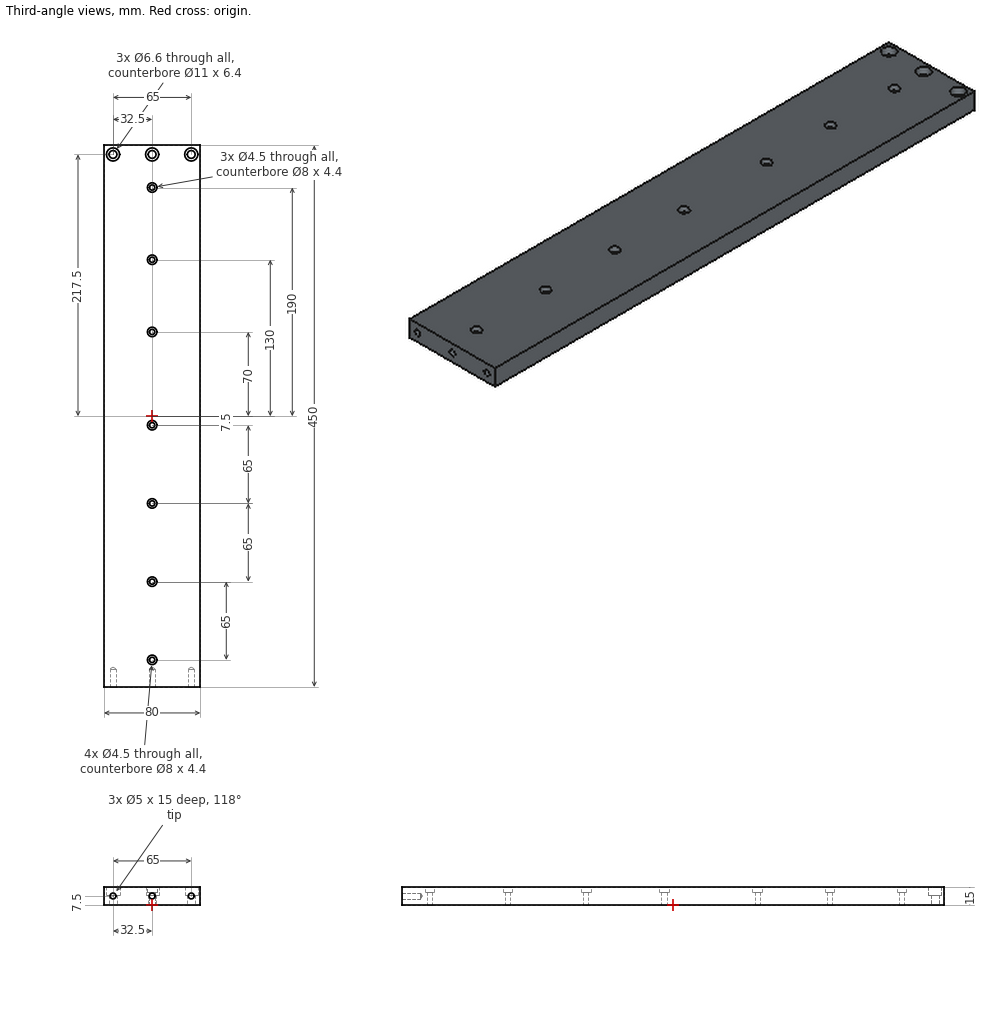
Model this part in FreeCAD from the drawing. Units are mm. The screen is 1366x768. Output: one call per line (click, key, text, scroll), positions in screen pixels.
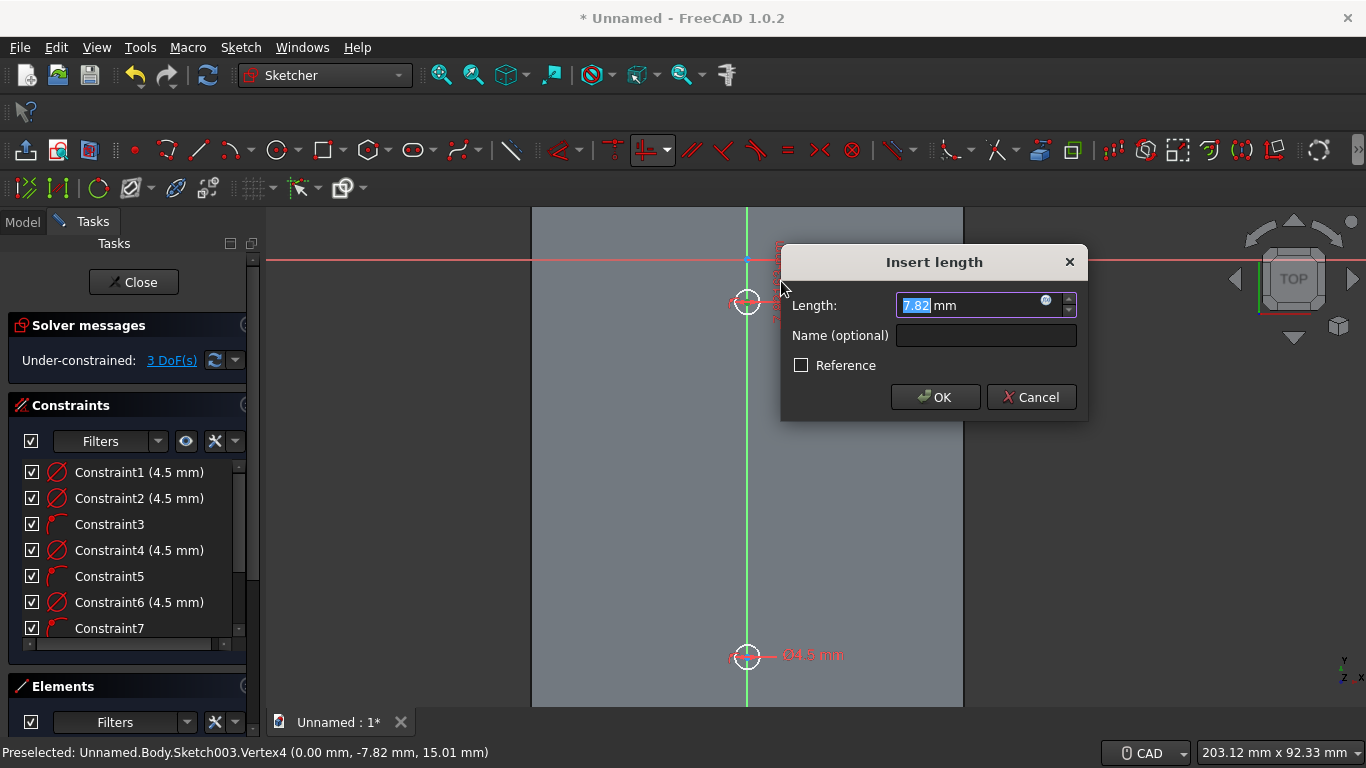
text(7.5)
key(Return)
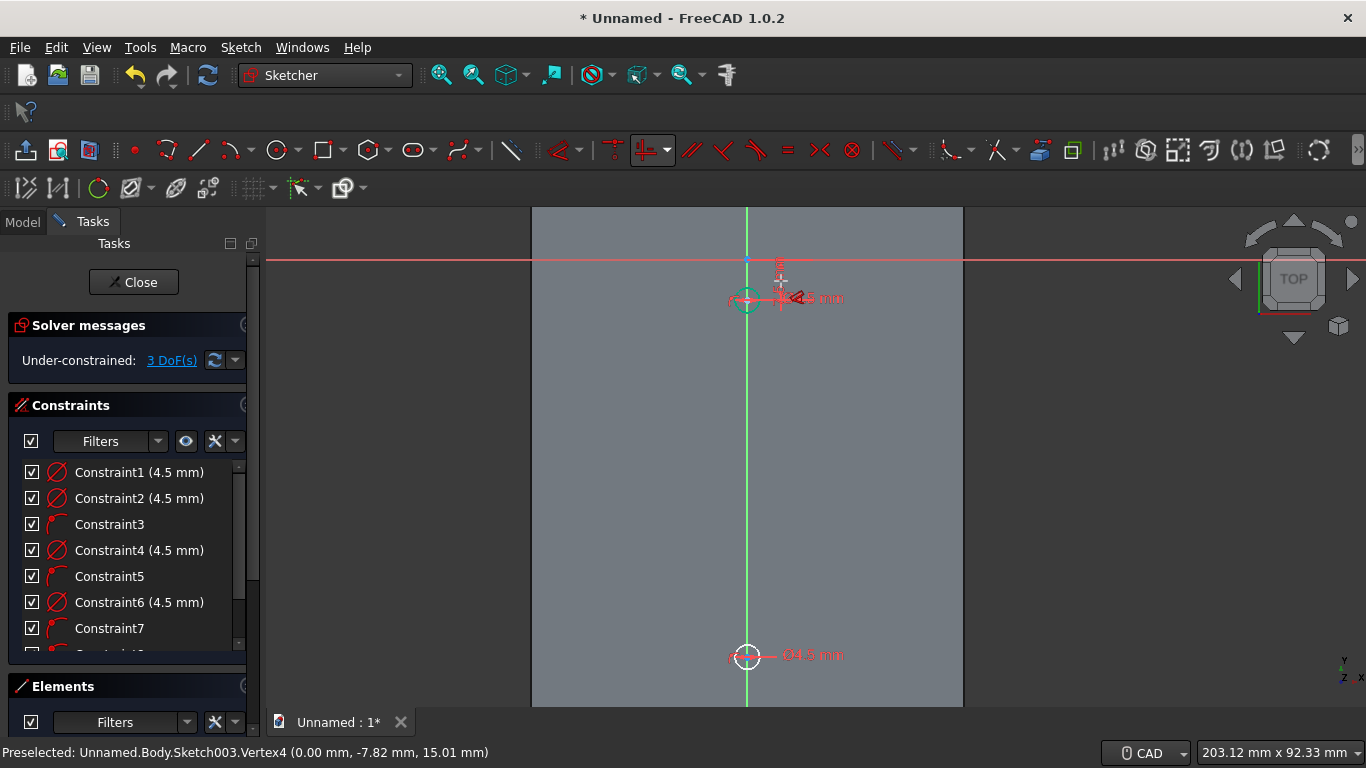
scroll(748, 303, down, 6)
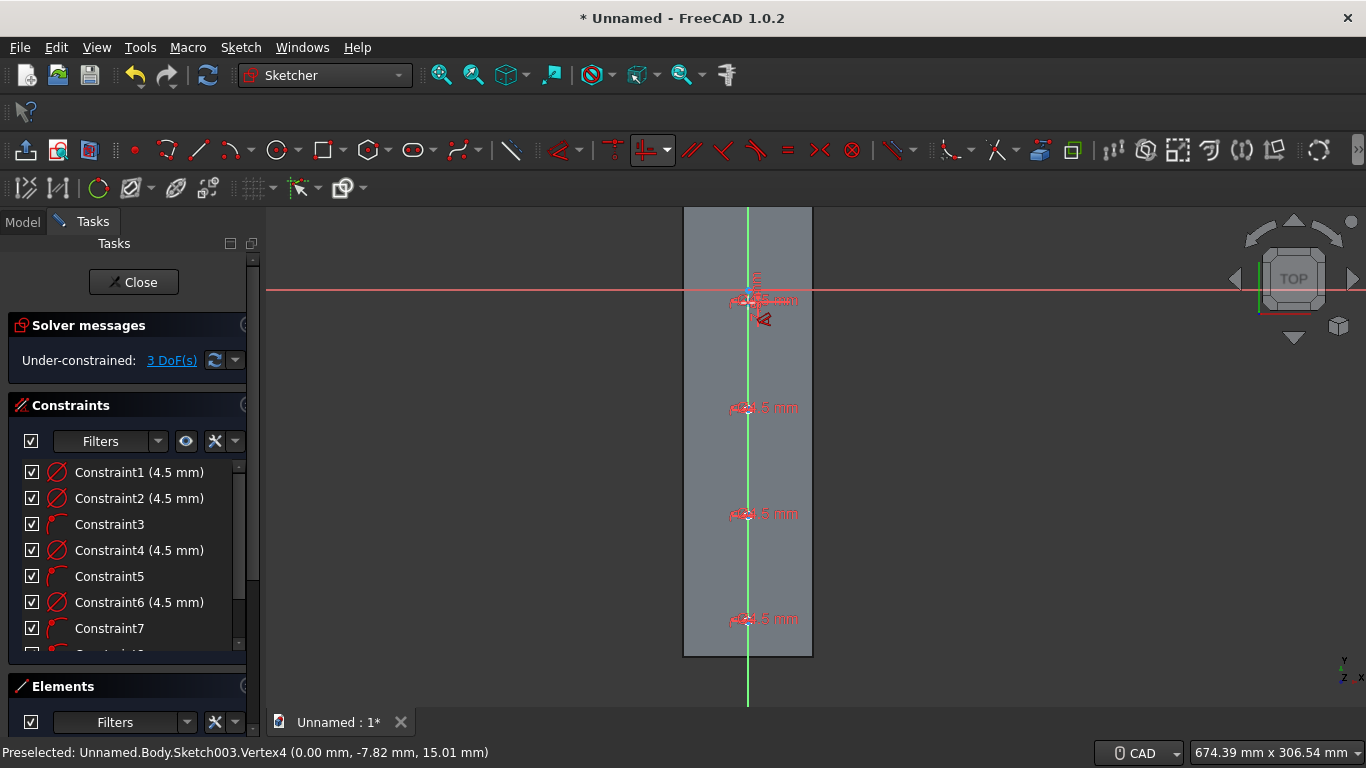
click(748, 621)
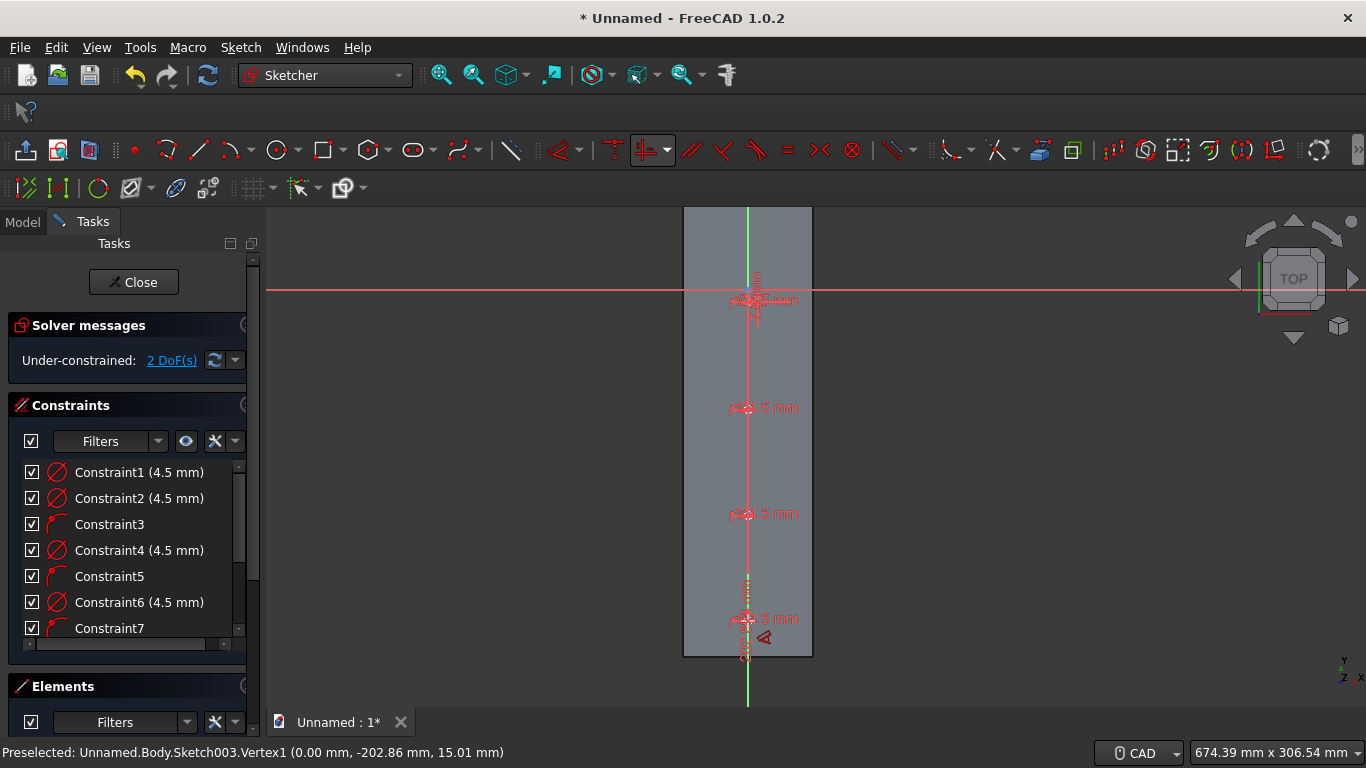
click(748, 516)
click(782, 568)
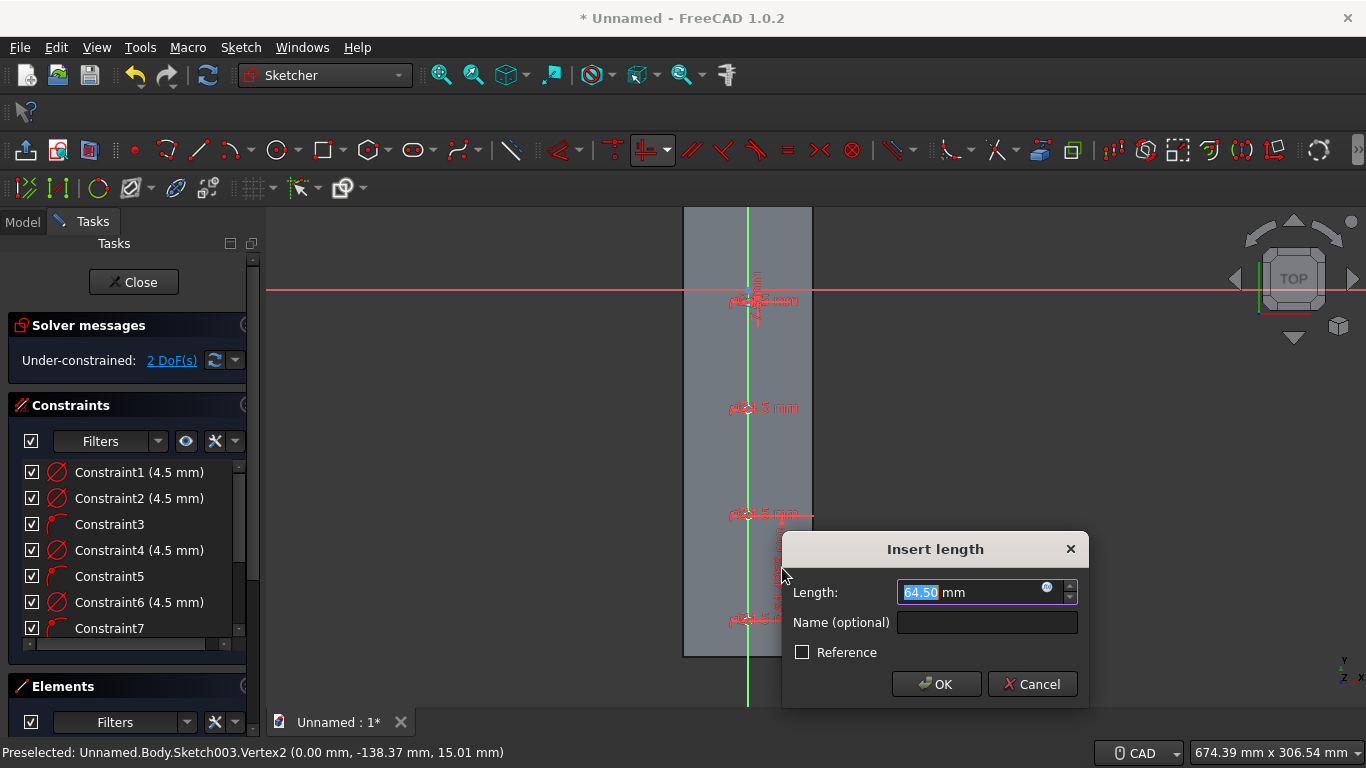
text(65)
key(Return)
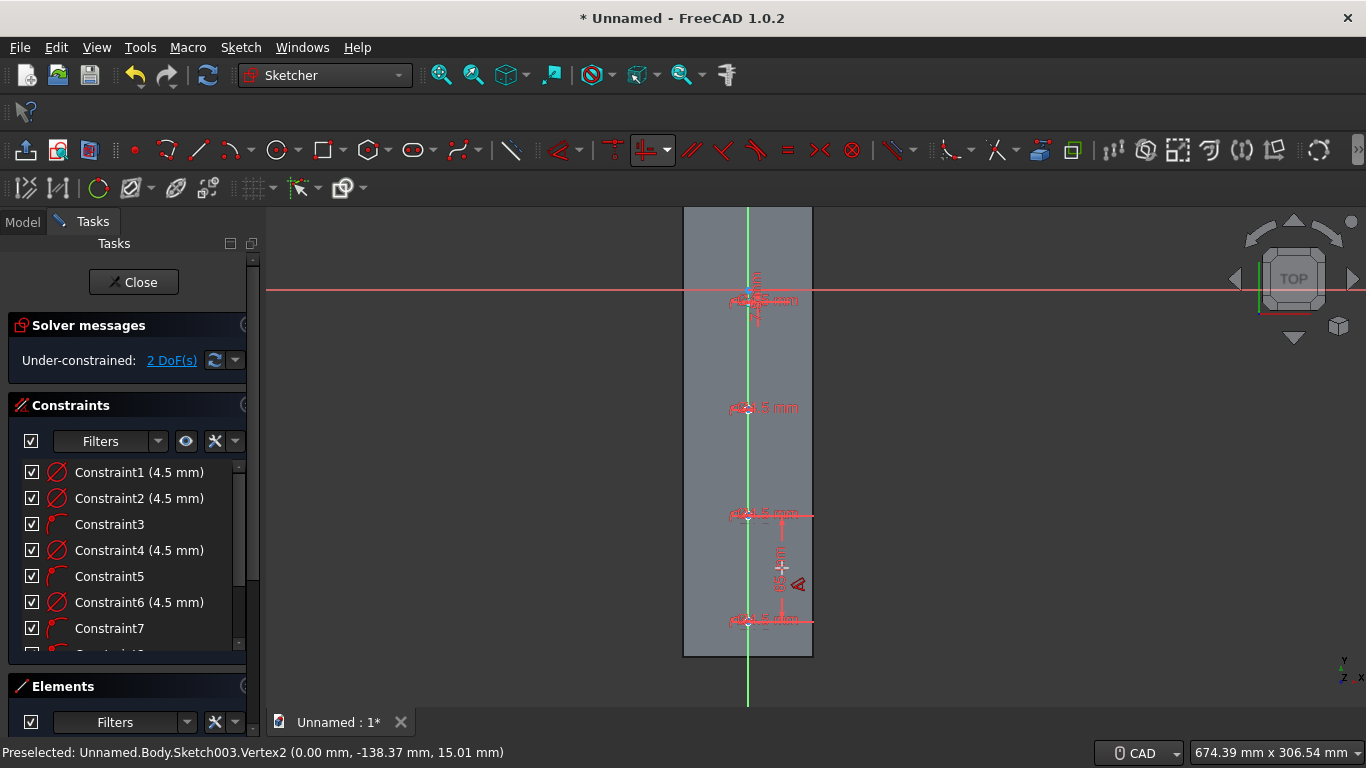
click(748, 516)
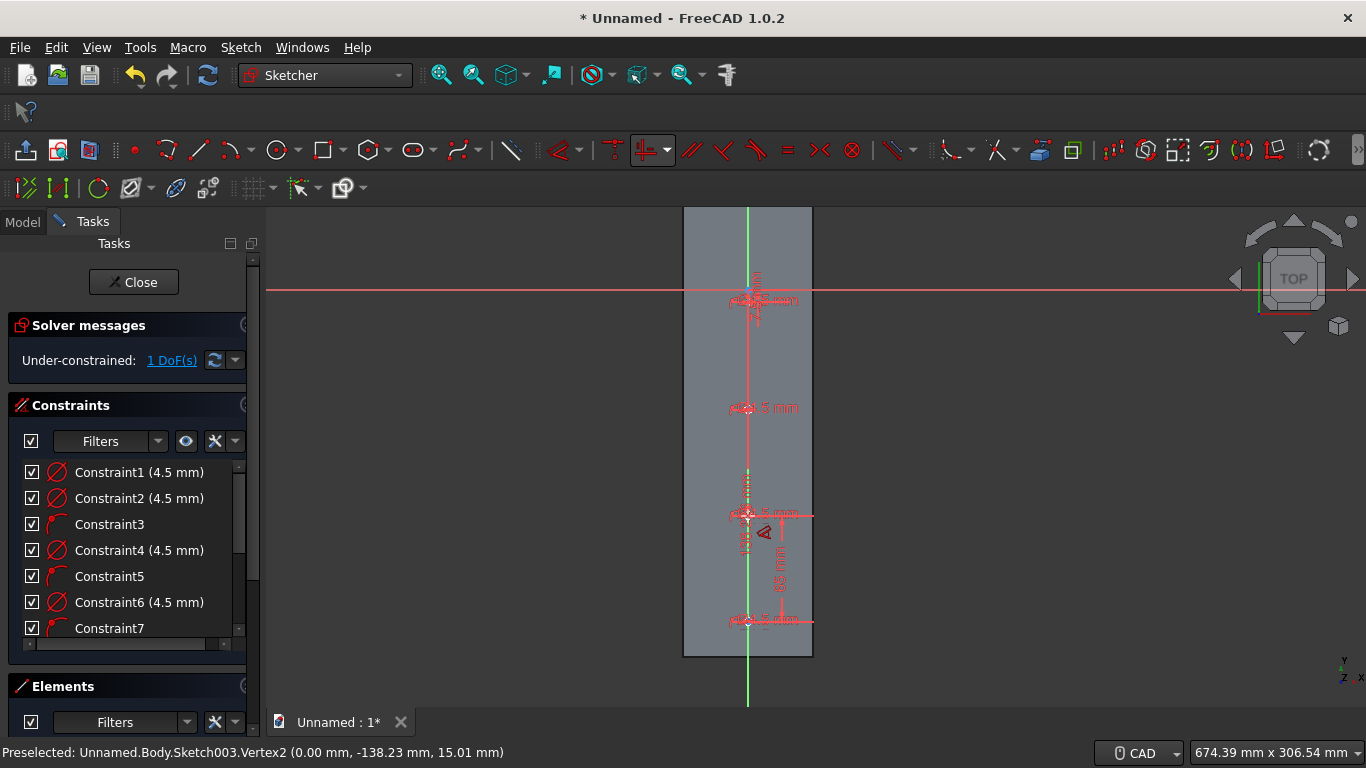
click(748, 410)
click(782, 463)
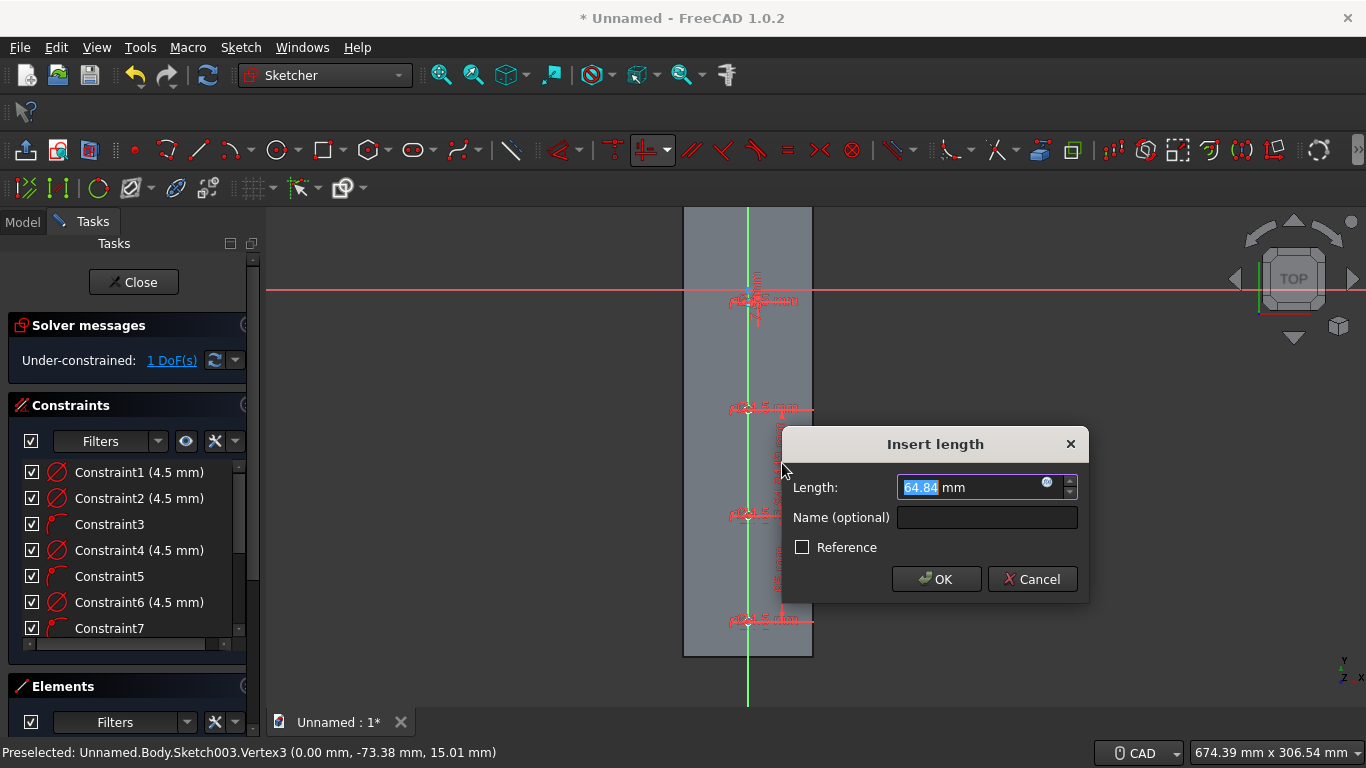
text(65)
key(Return)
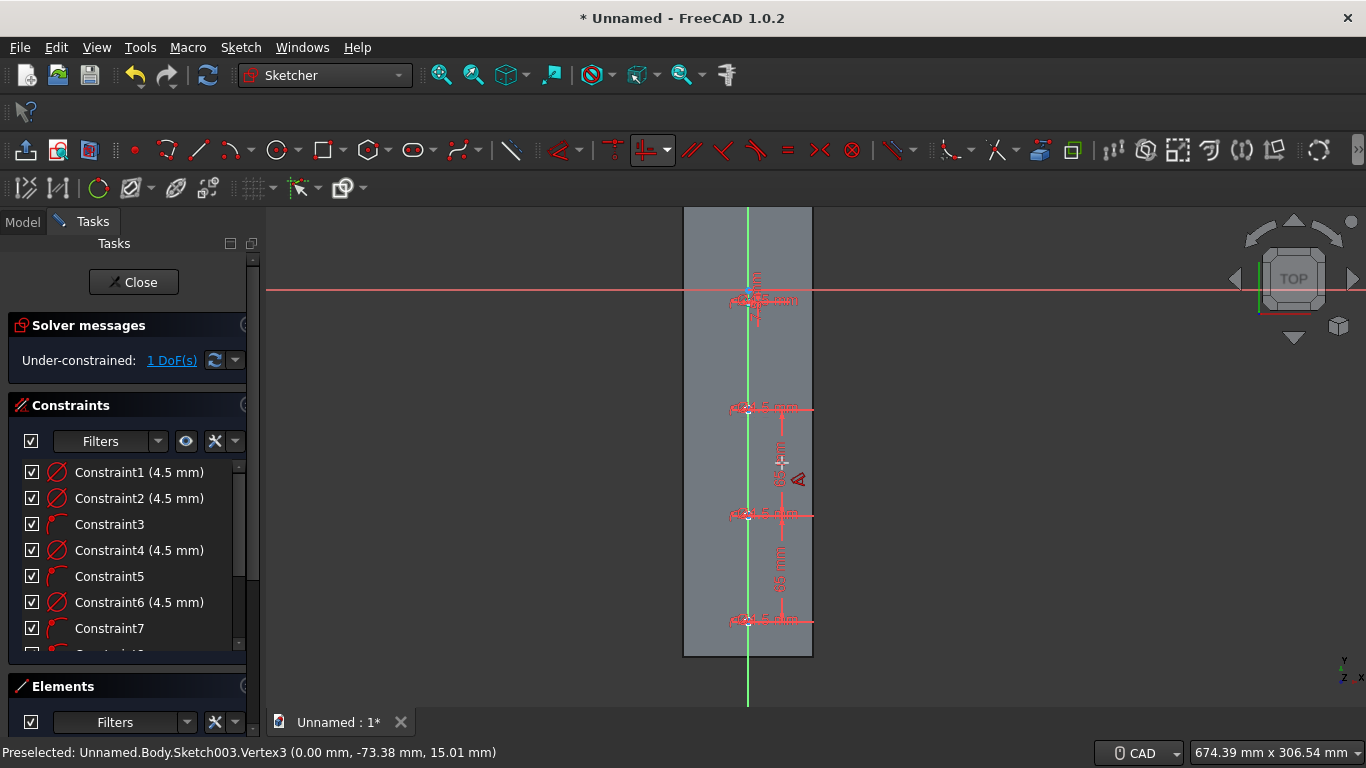
click(748, 410)